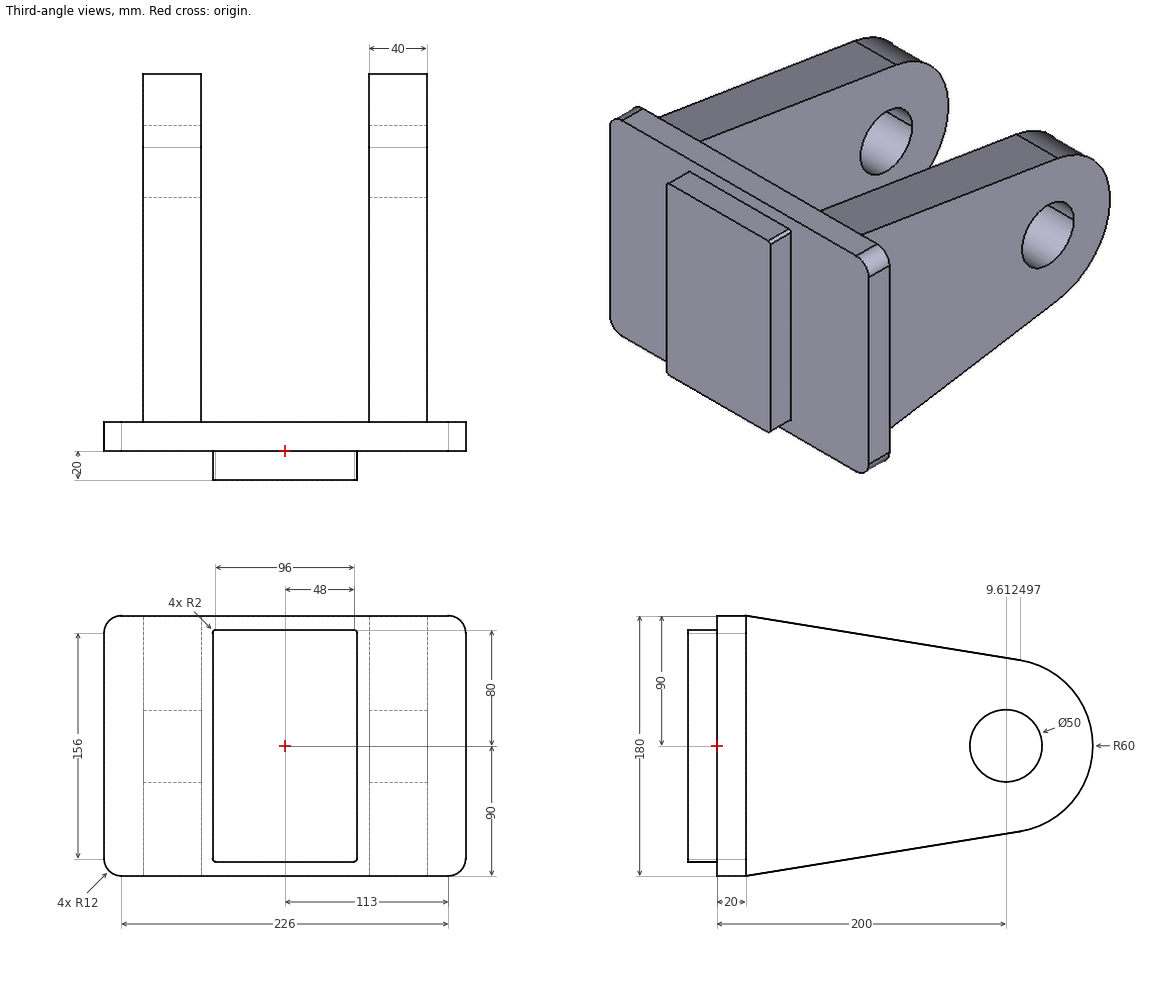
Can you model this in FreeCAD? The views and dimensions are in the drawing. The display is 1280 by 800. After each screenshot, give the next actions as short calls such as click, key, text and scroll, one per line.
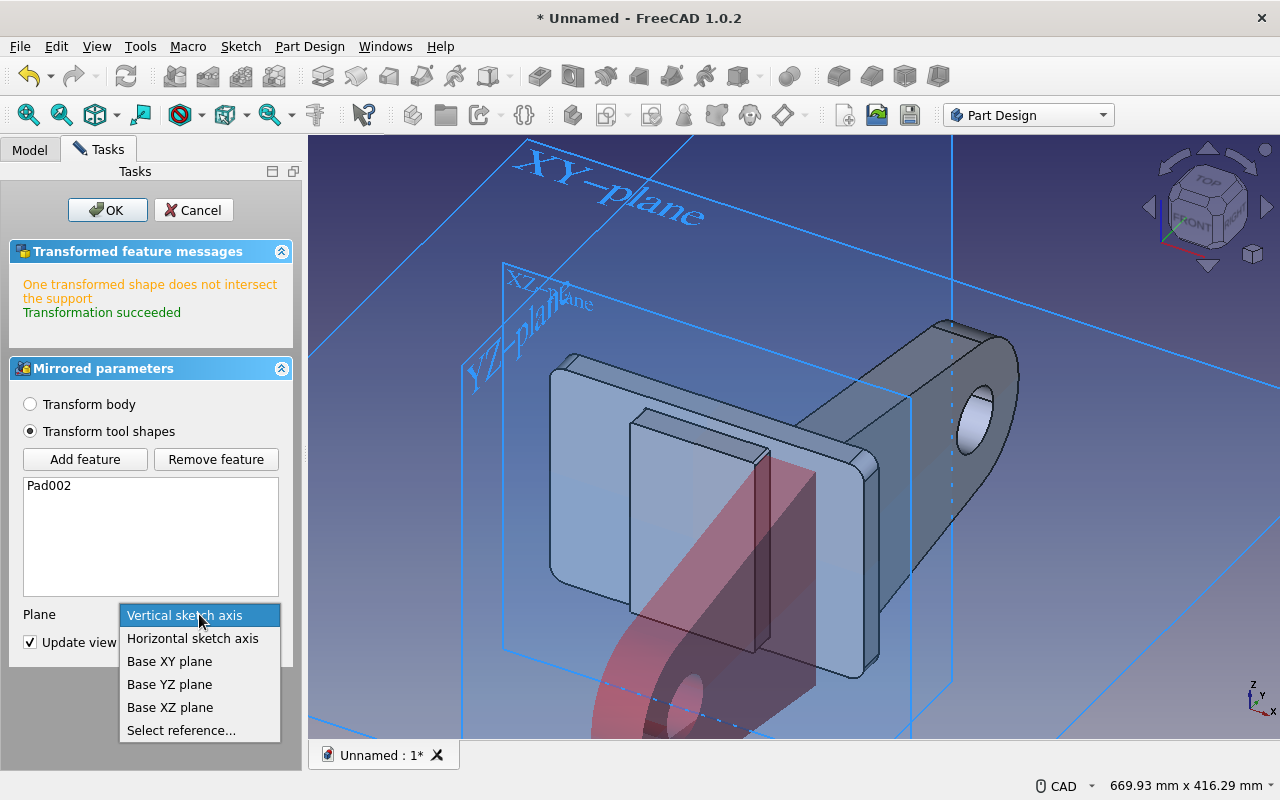
click(198, 684)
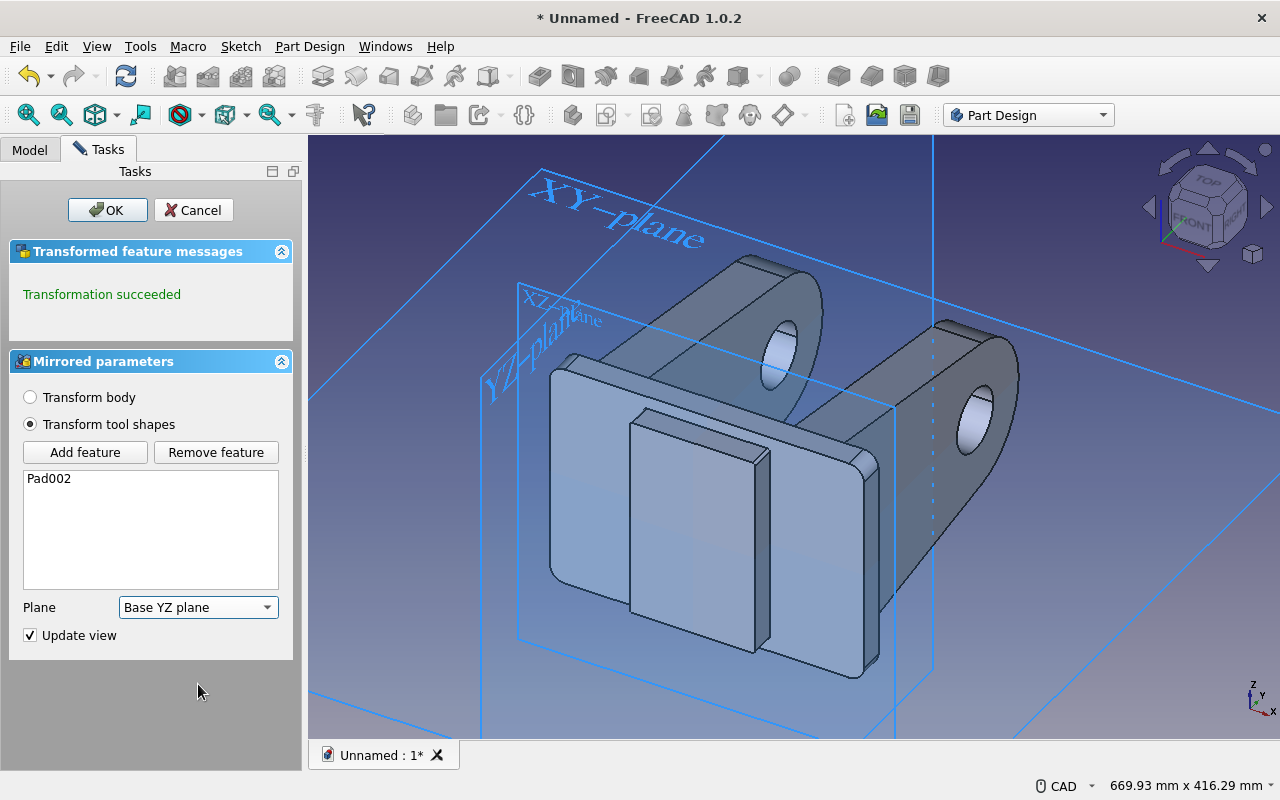
click(108, 210)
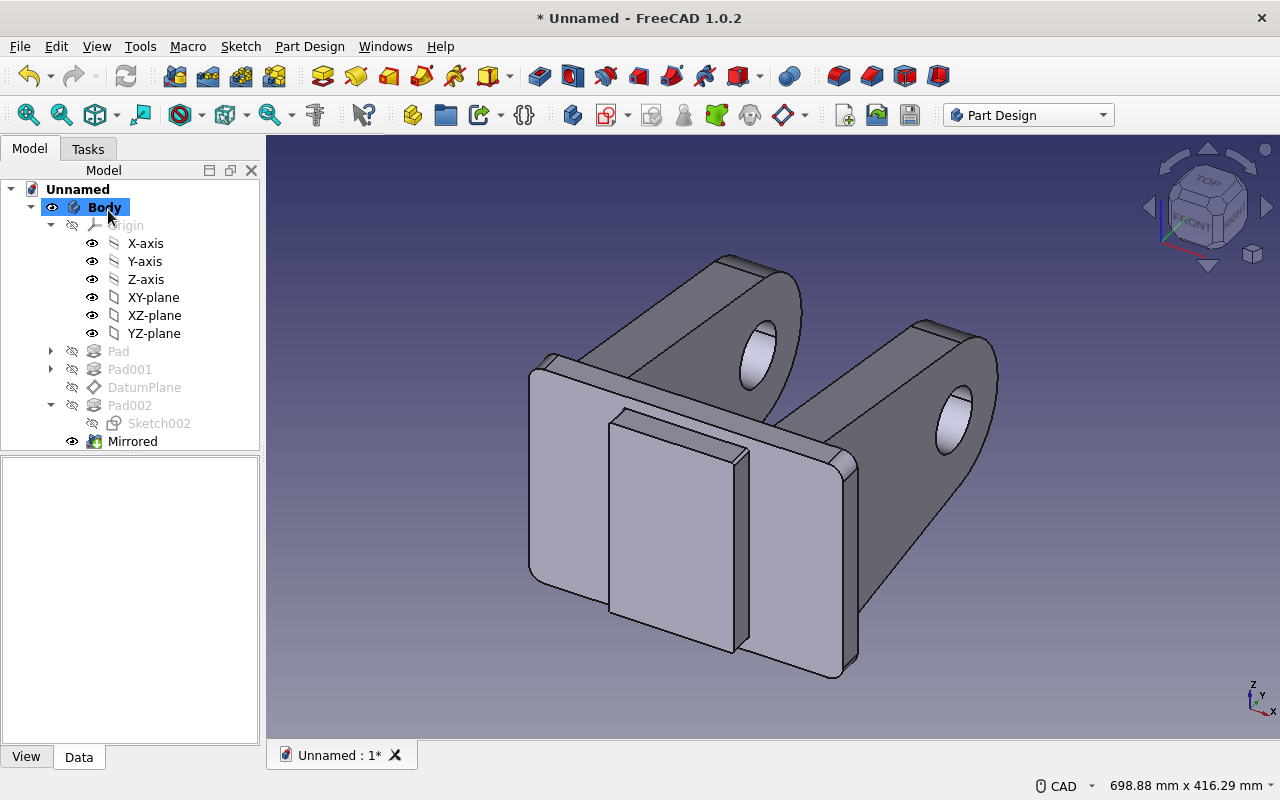
key(0)